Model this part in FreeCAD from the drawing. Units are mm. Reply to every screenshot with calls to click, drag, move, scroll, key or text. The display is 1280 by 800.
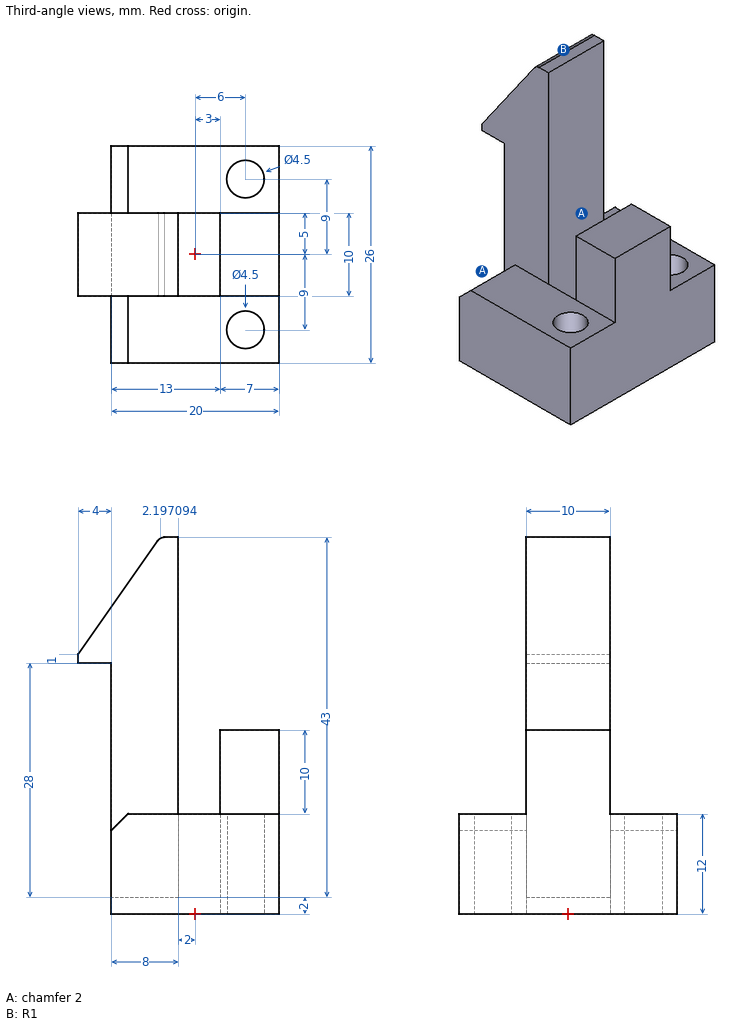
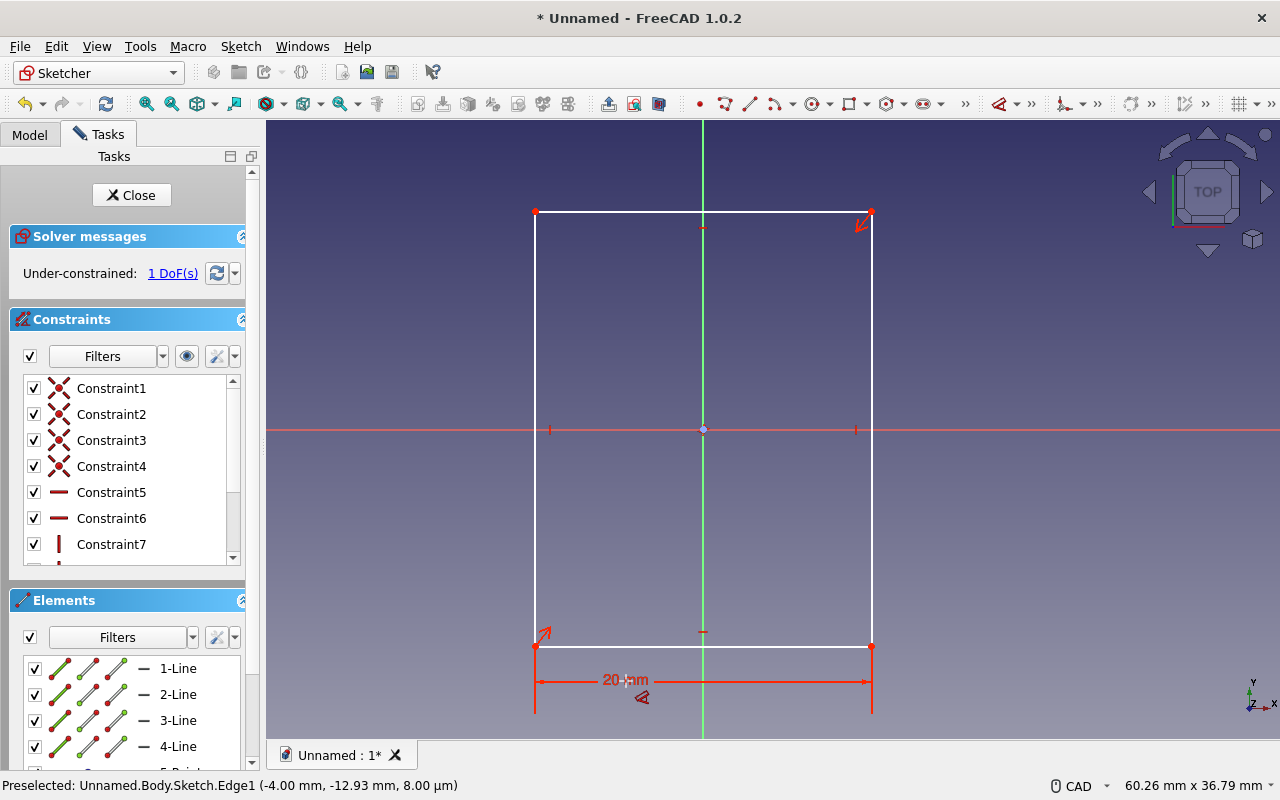
click(872, 517)
click(906, 329)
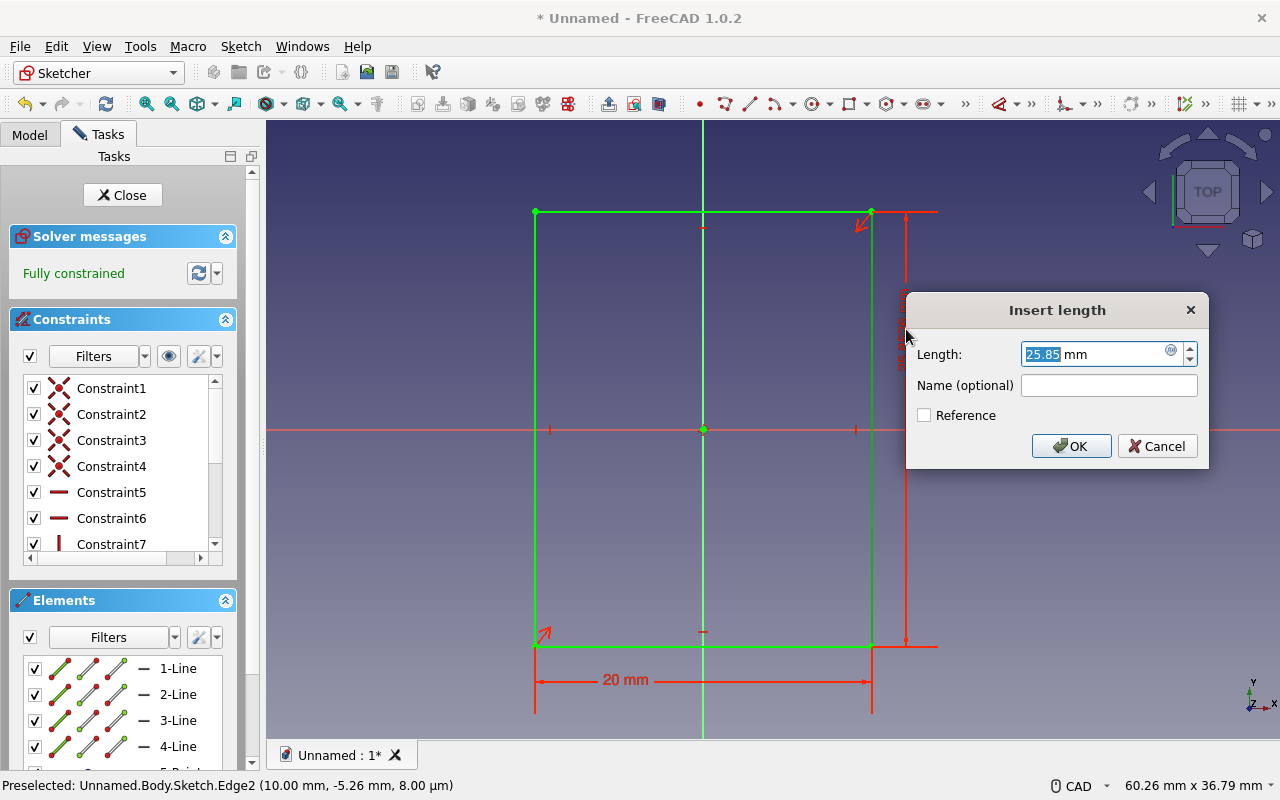
text(26)
key(Return)
key(Escape)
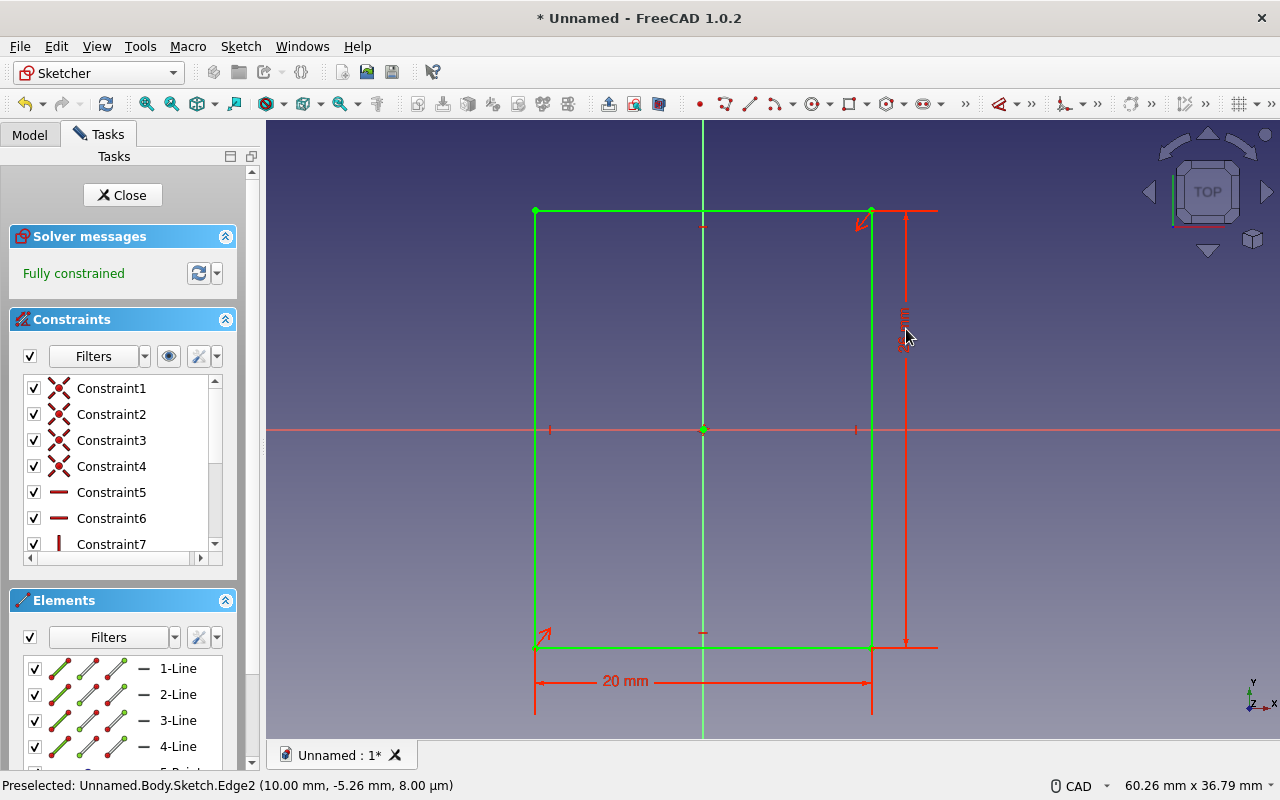
click(123, 195)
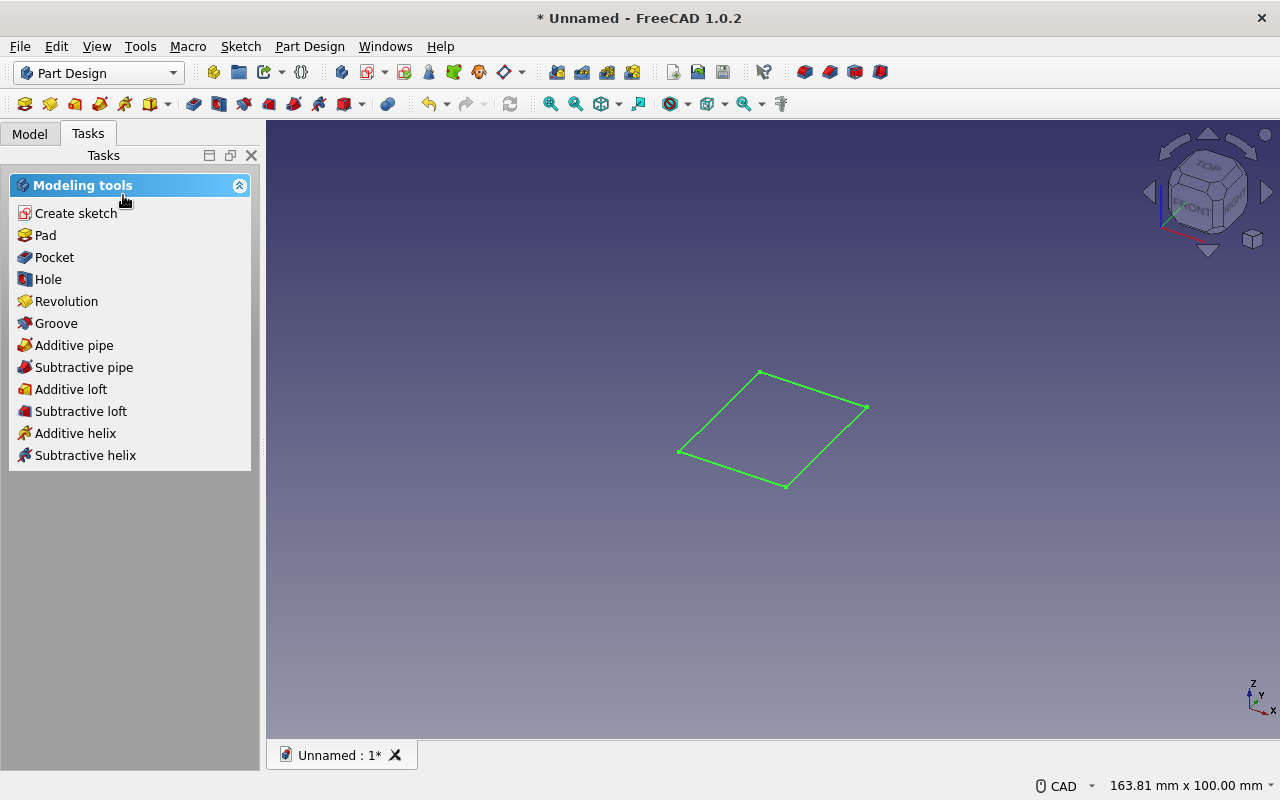
click(25, 104)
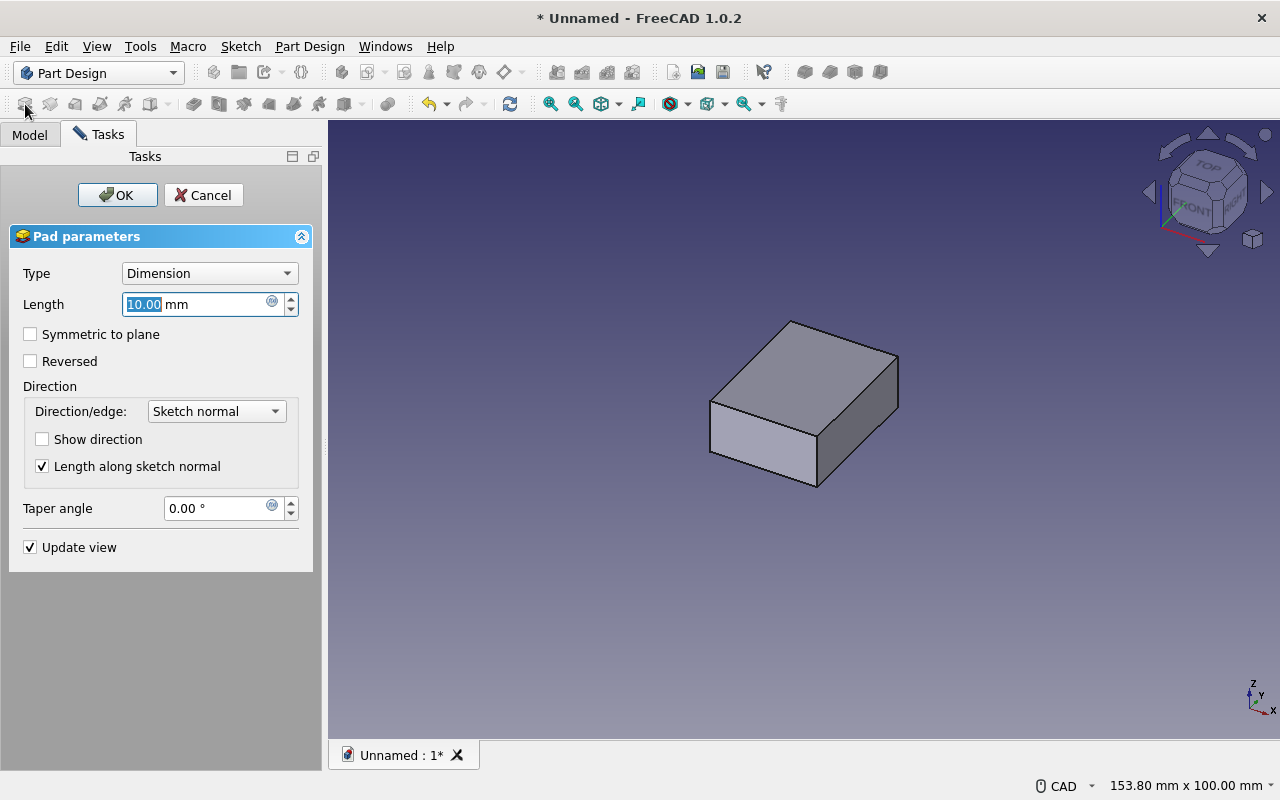
text(12)
key(Tab)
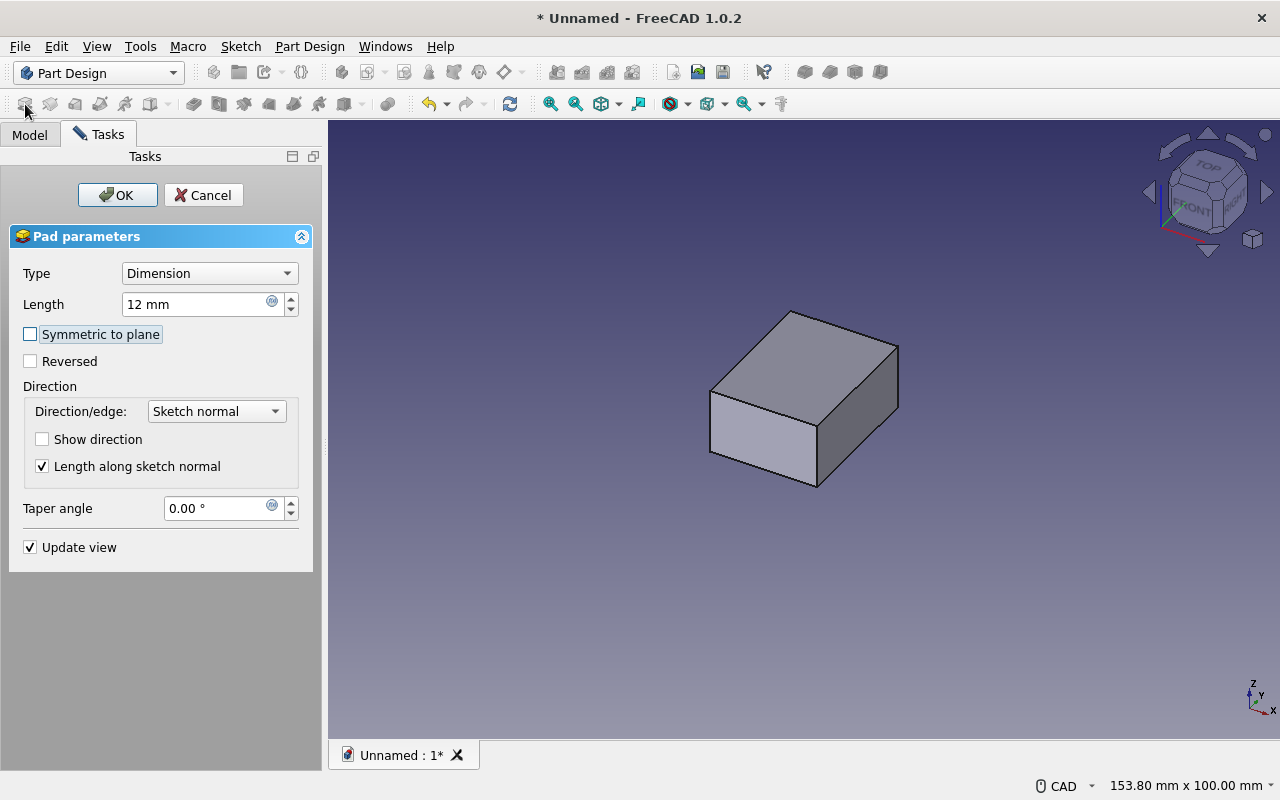
click(118, 195)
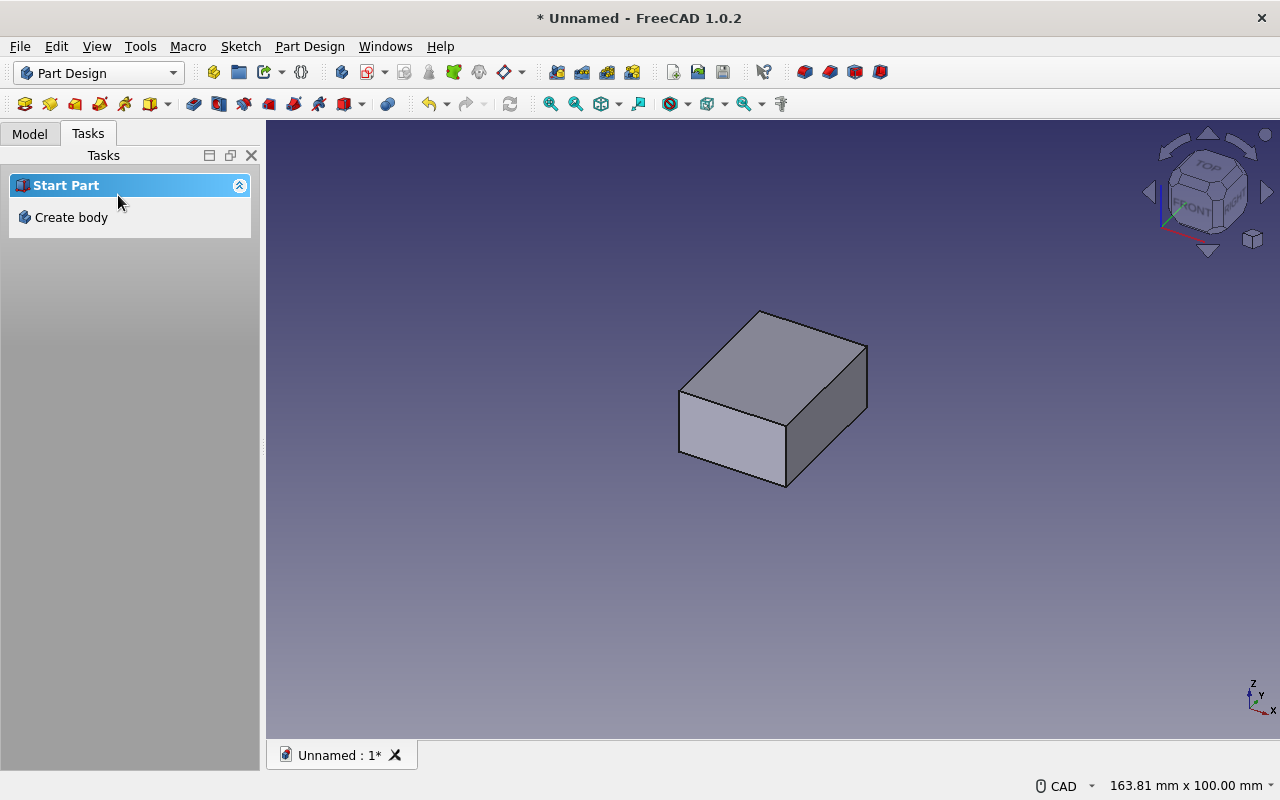
key(v)
key(f)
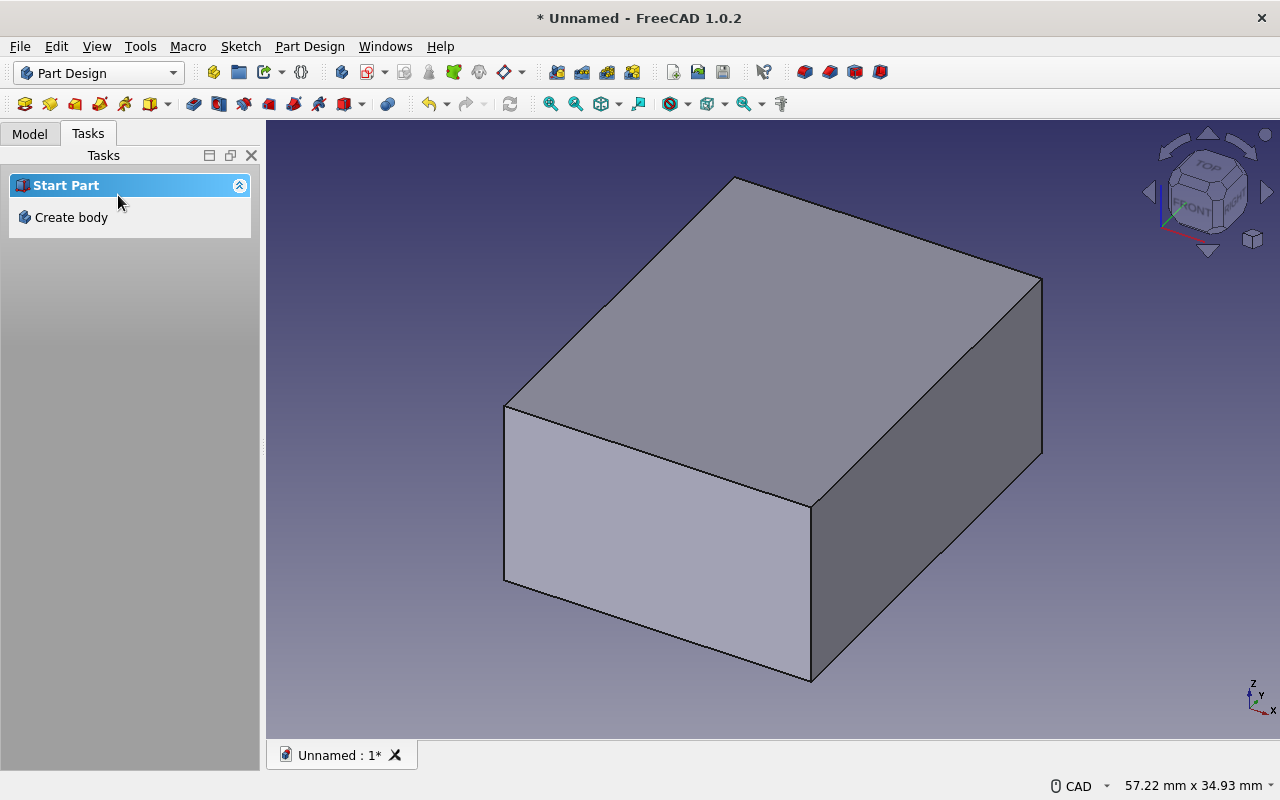
click(773, 341)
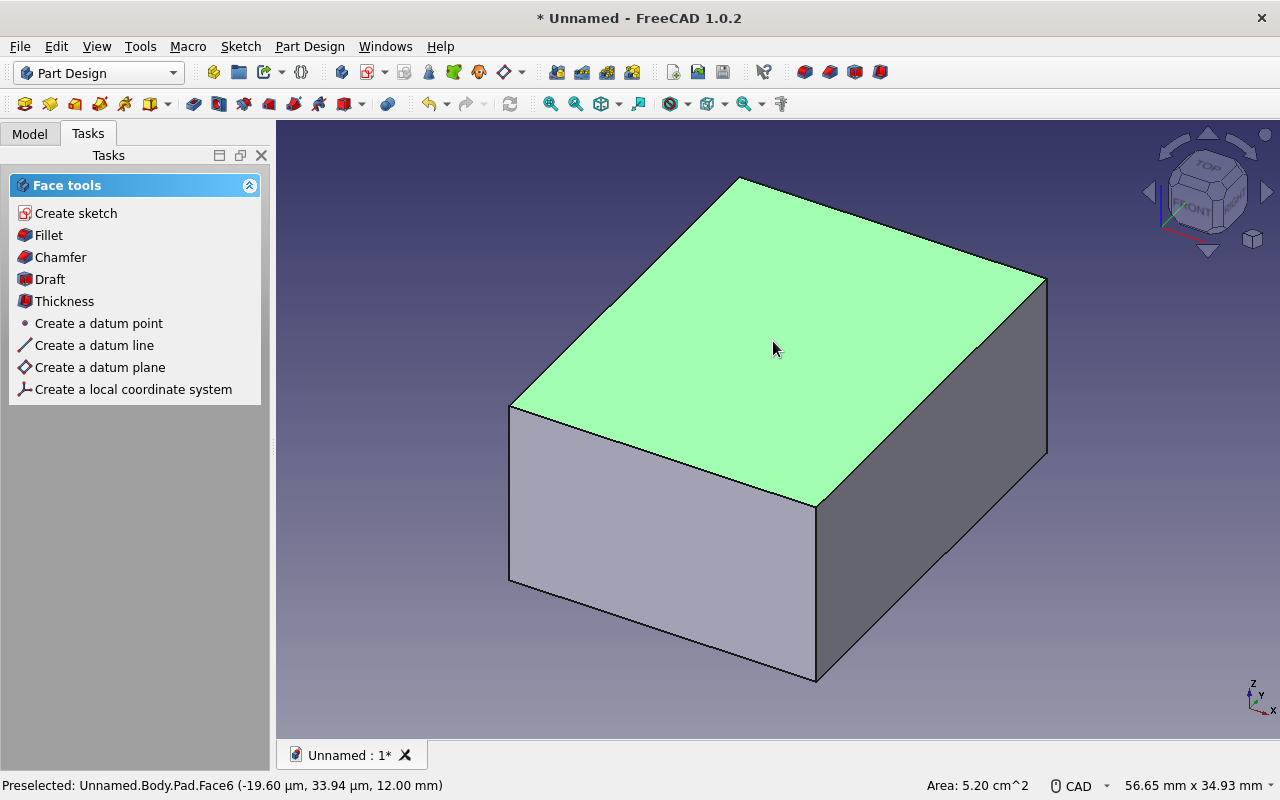
click(366, 72)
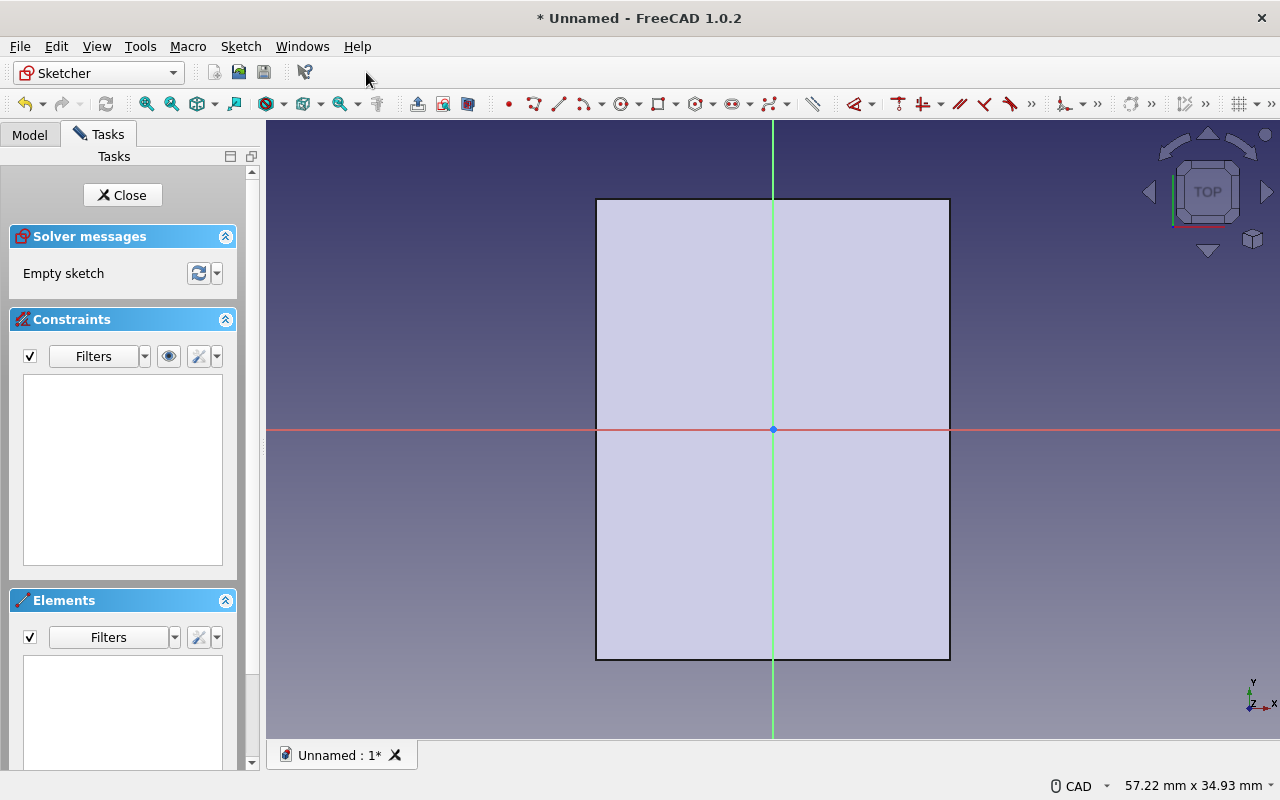
scroll(924, 230, up, 8)